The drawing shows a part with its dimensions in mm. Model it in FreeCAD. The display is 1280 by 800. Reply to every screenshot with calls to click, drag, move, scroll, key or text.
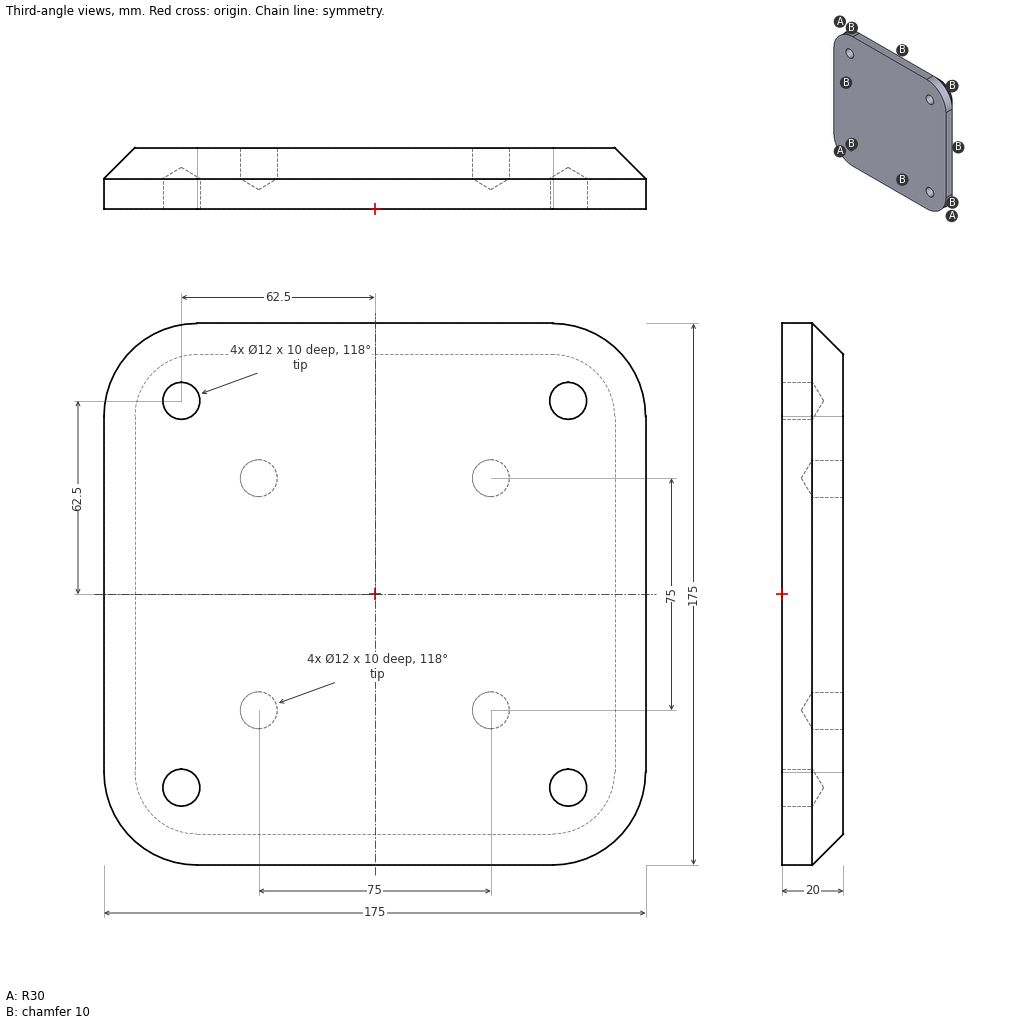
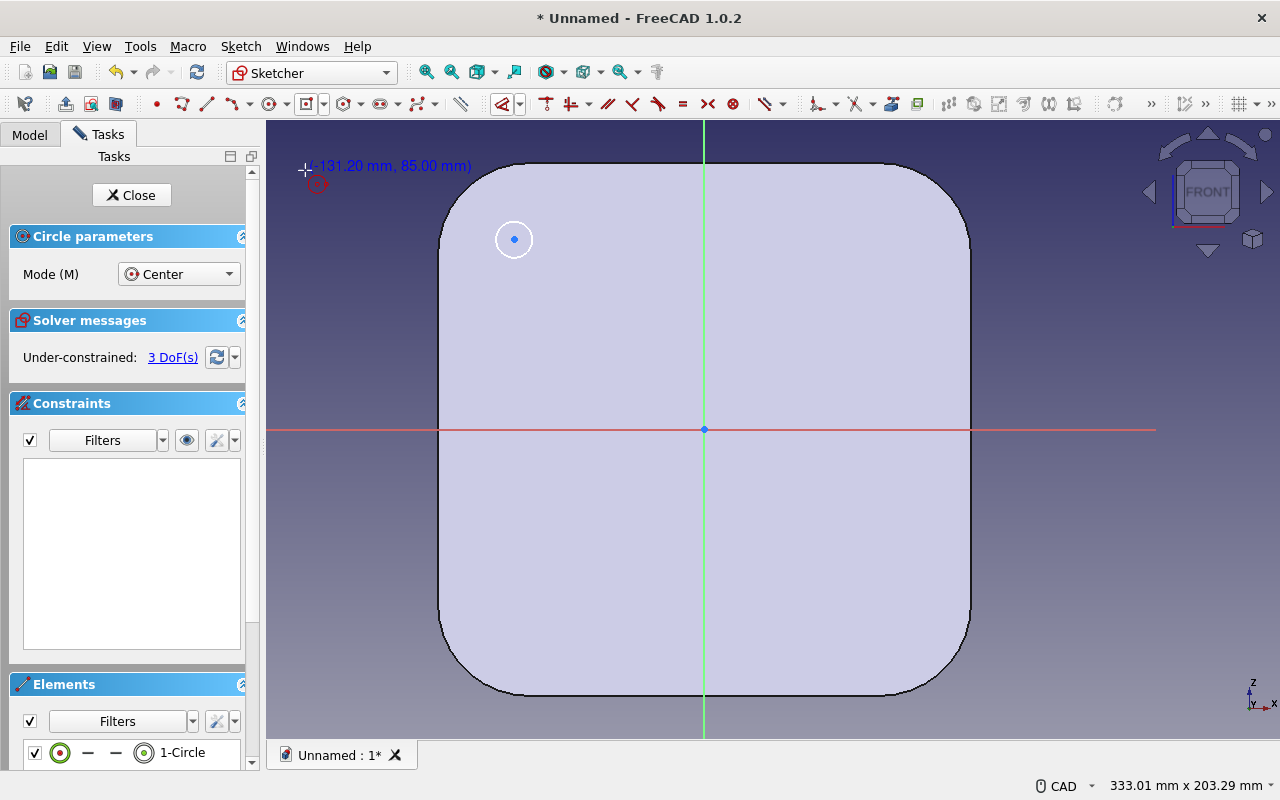
scroll(895, 239, up, 2)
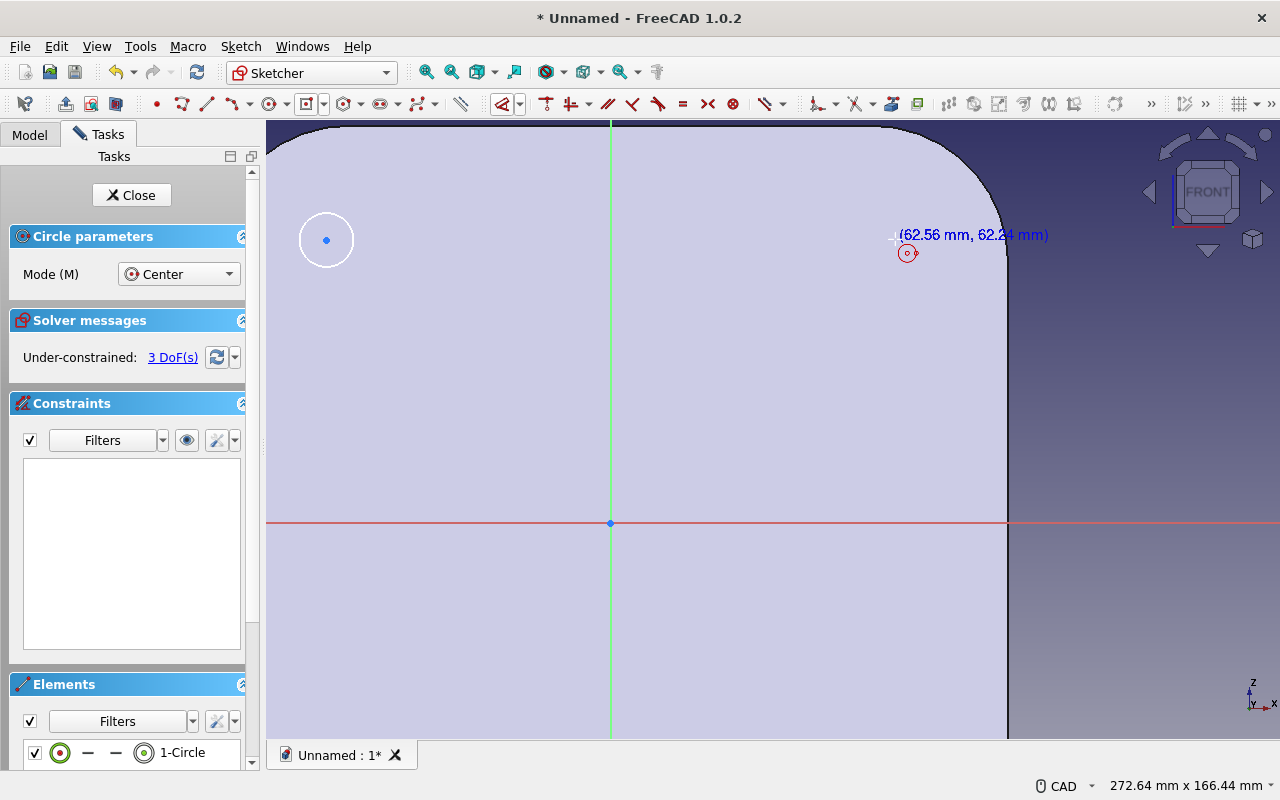
click(894, 239)
click(914, 220)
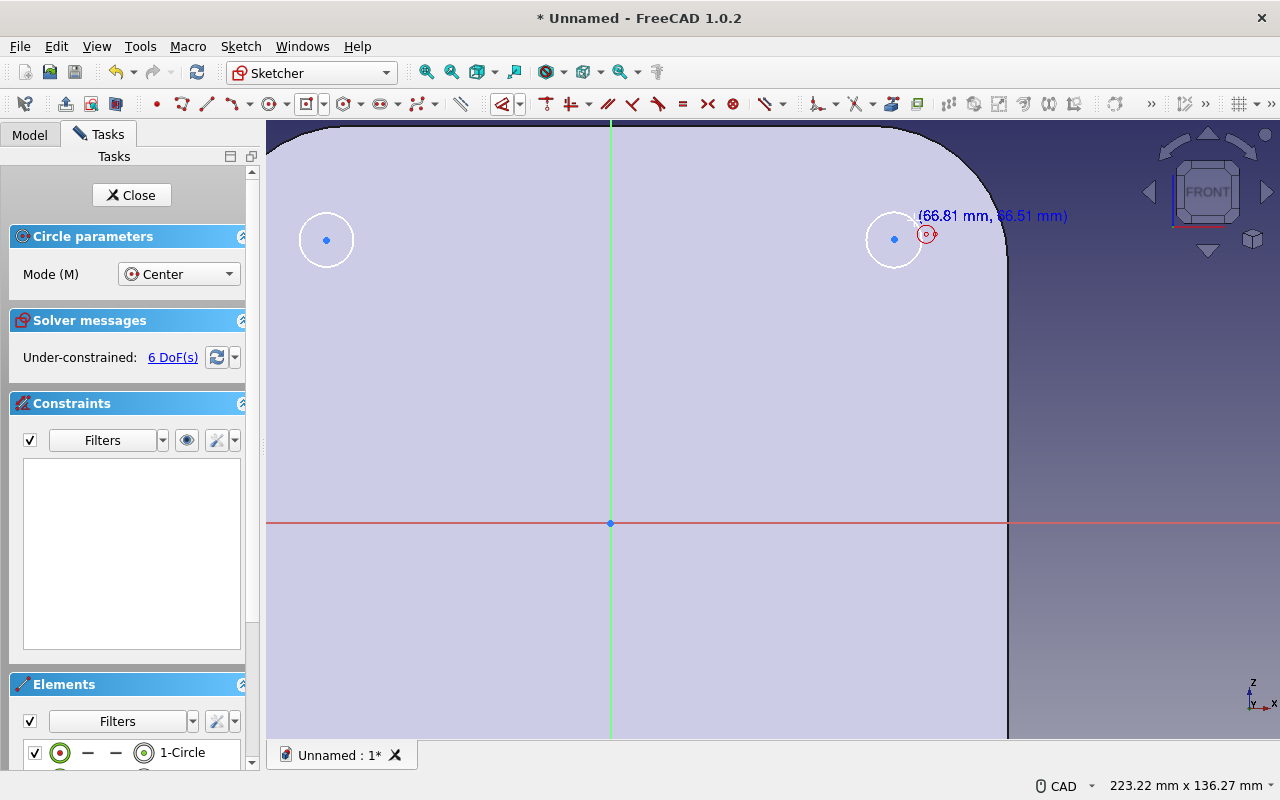
scroll(896, 239, down, 2)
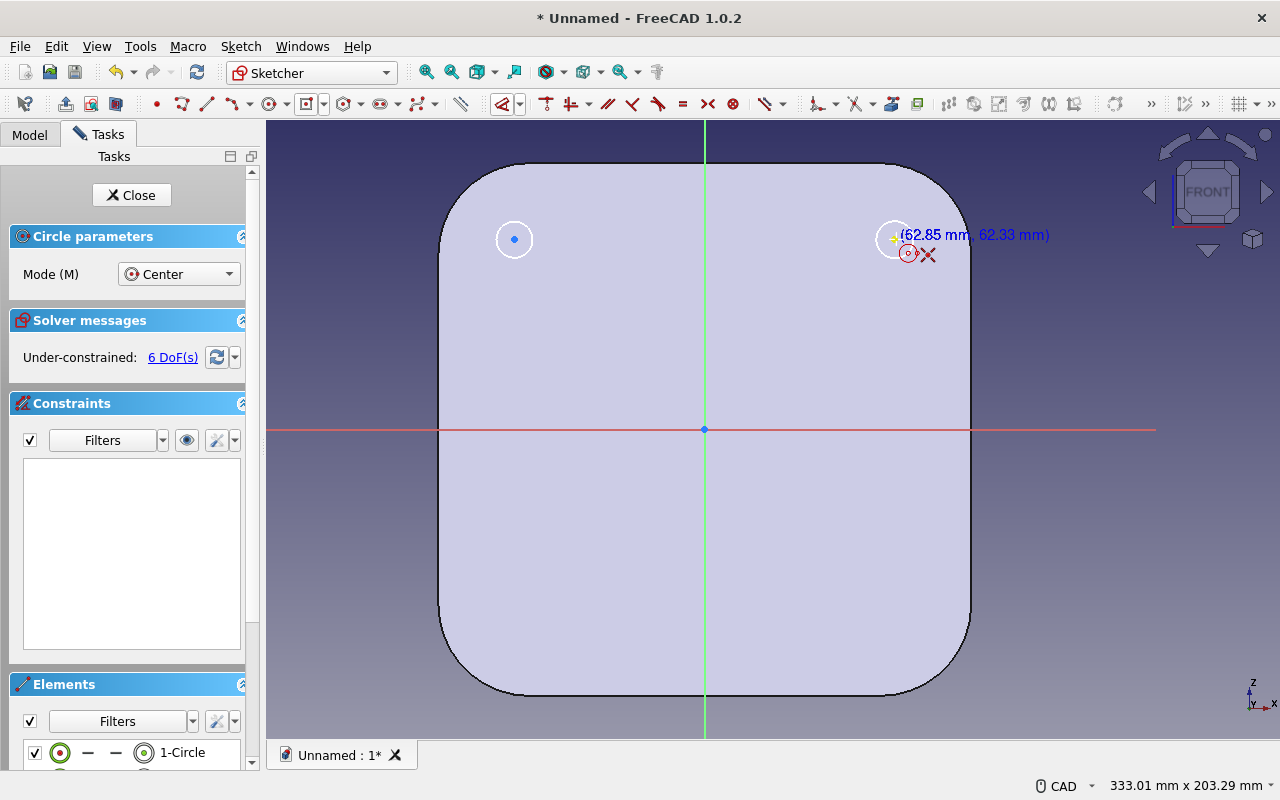
scroll(895, 620, up, 2)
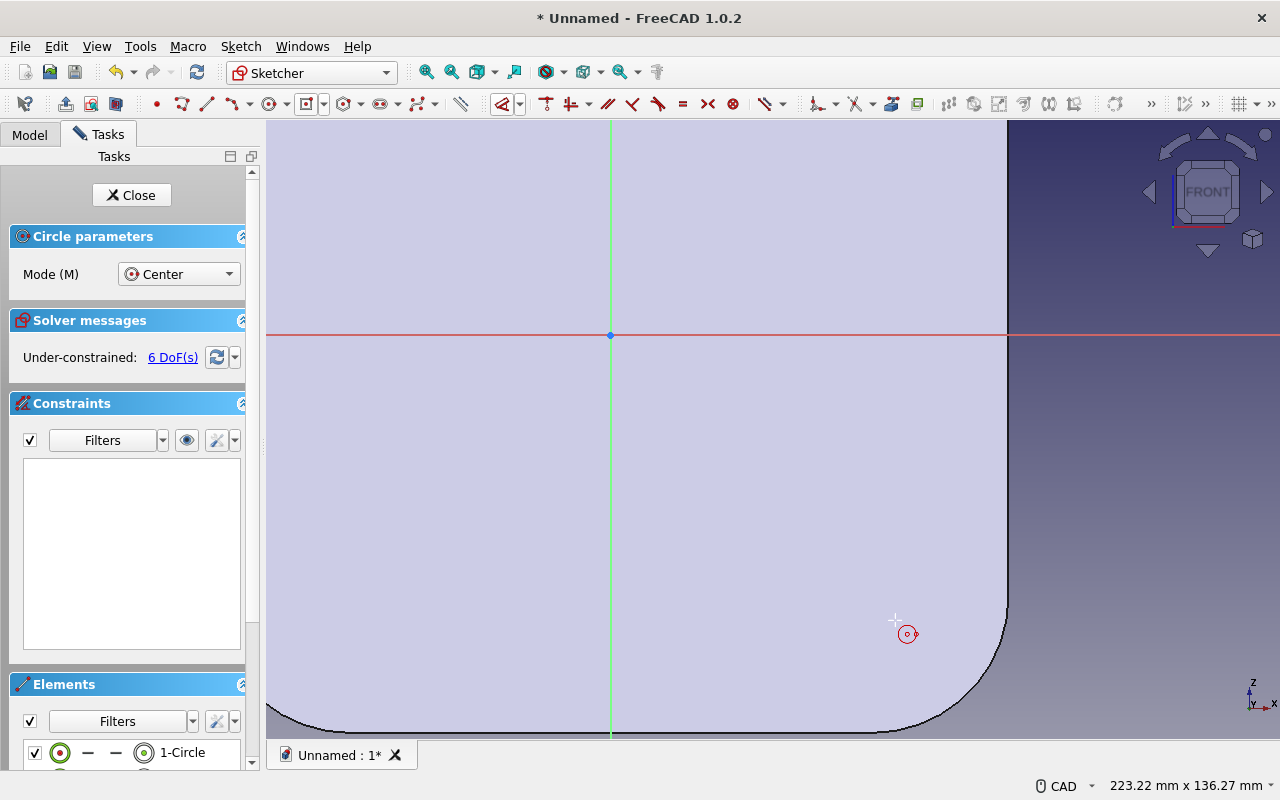
click(895, 619)
click(914, 600)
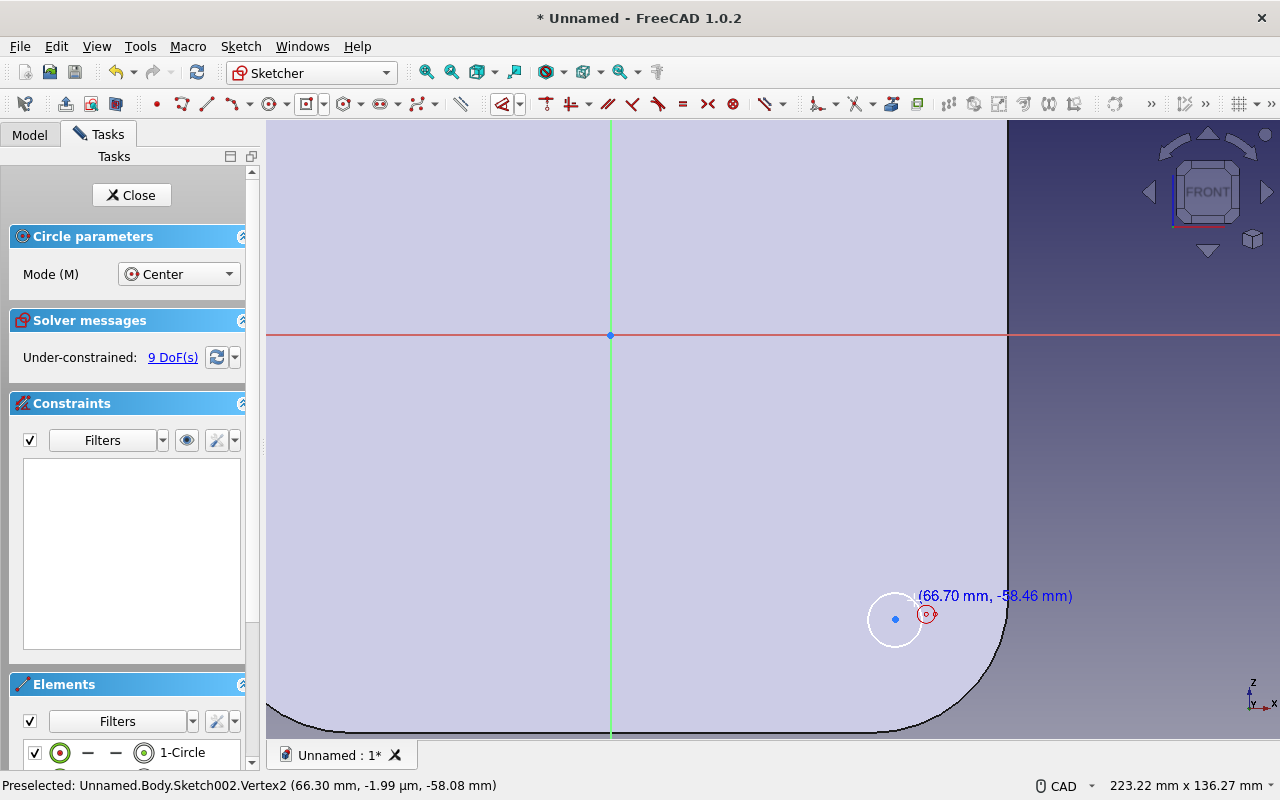
click(327, 619)
click(346, 600)
key(Escape)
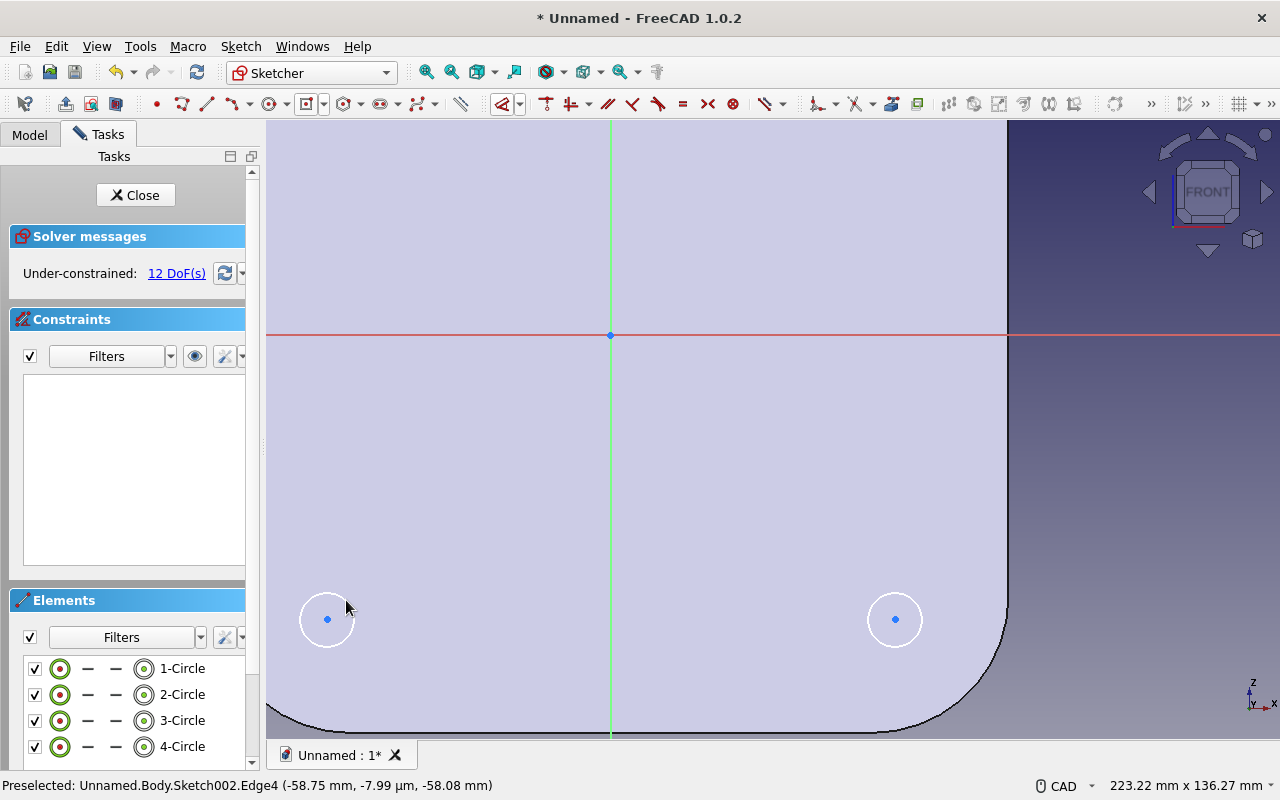
scroll(895, 621, down, 2)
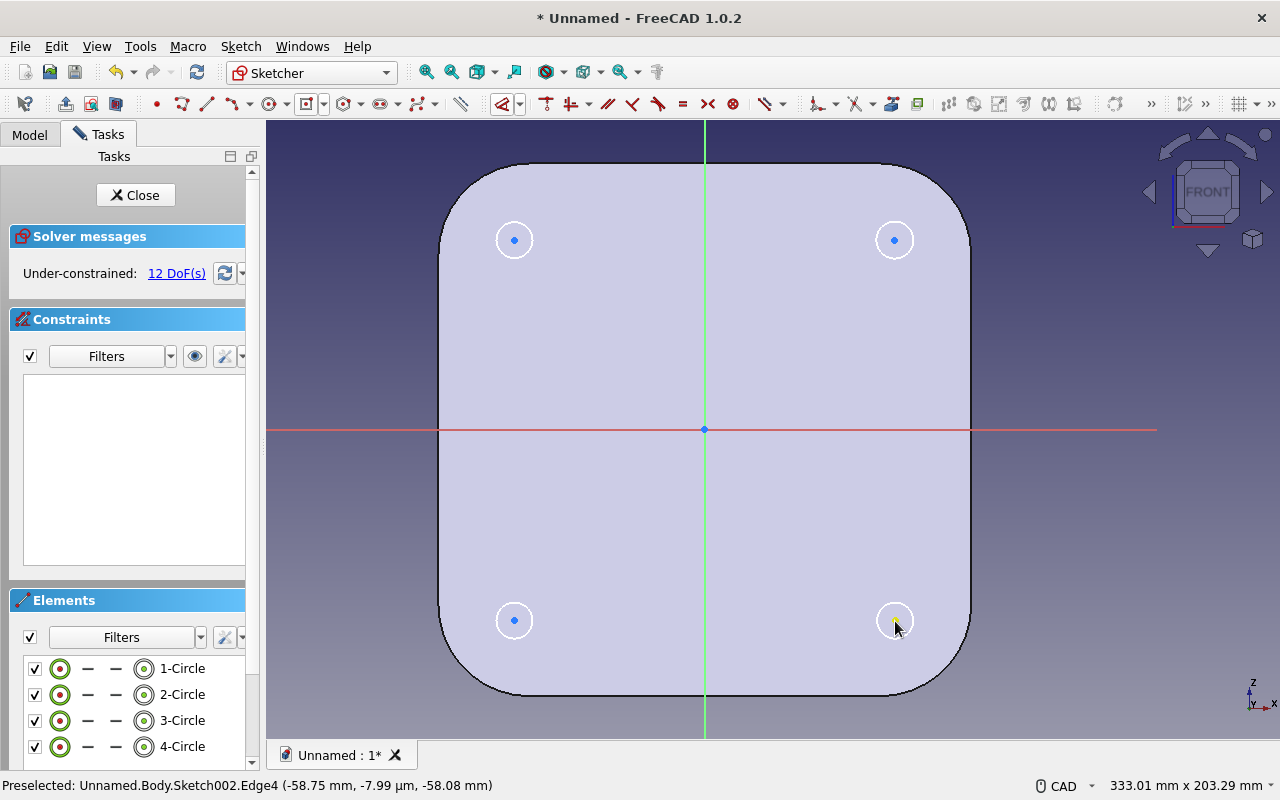
click(527, 227)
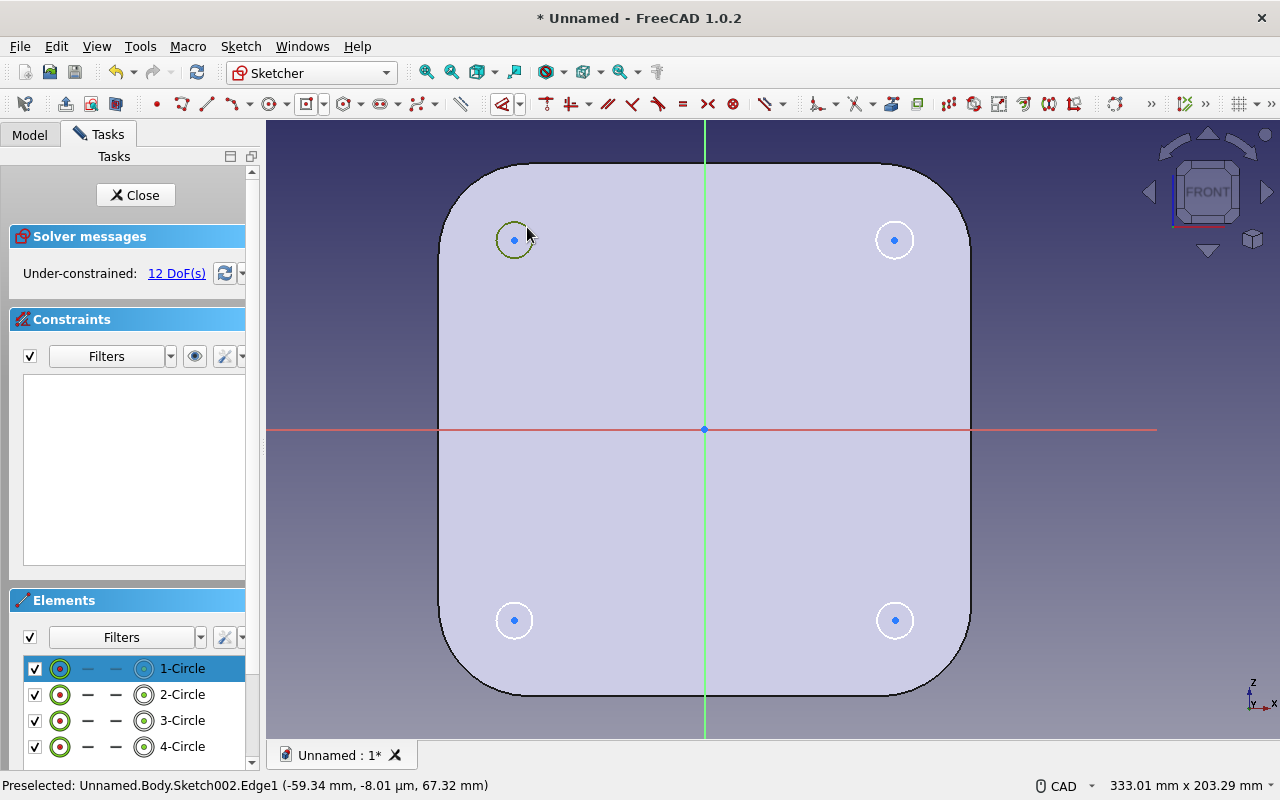
click(908, 227)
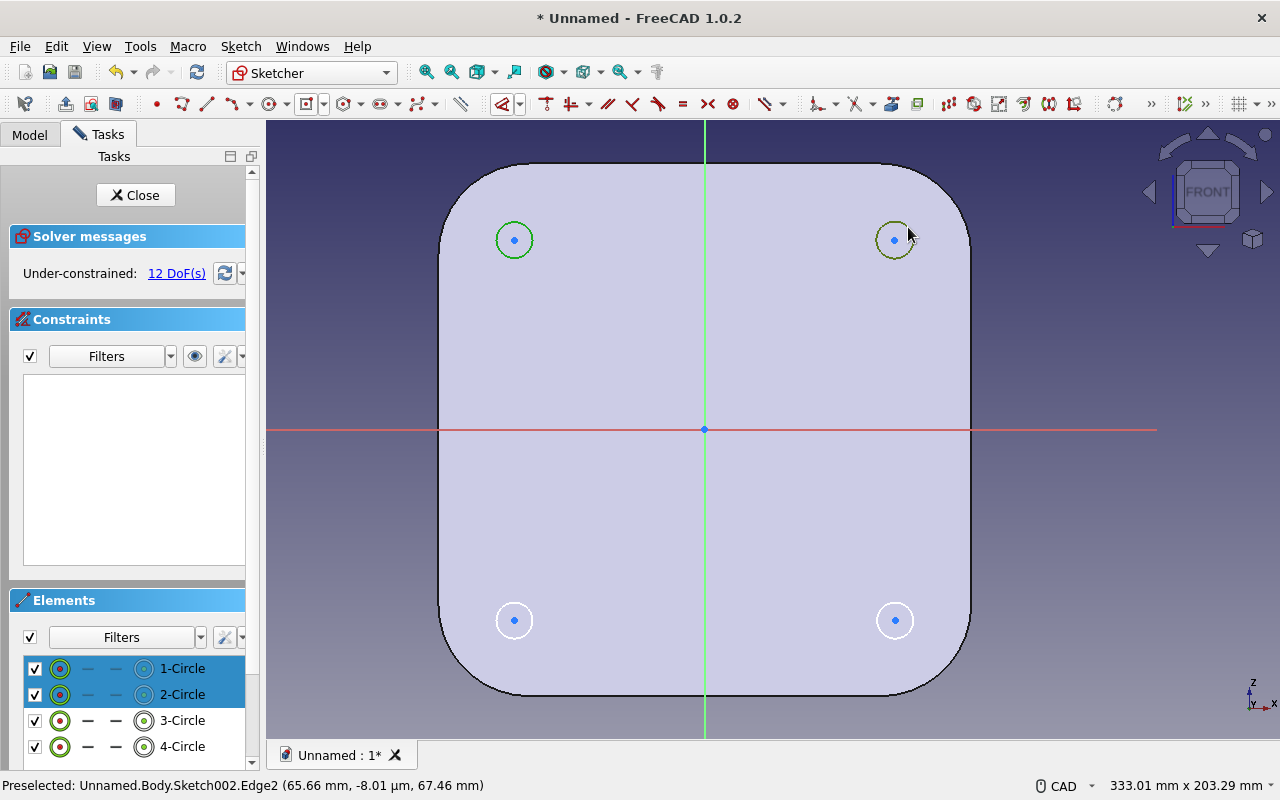
click(908, 608)